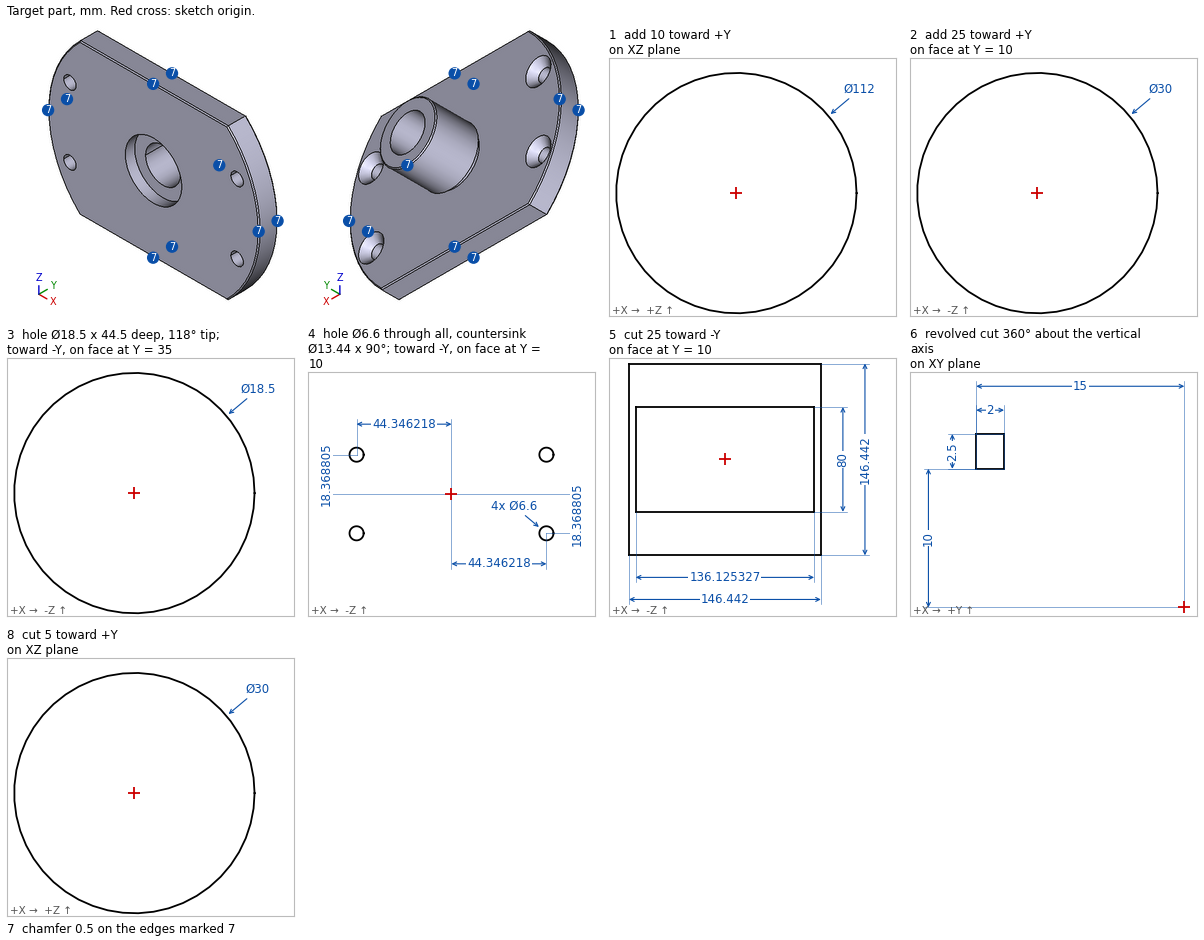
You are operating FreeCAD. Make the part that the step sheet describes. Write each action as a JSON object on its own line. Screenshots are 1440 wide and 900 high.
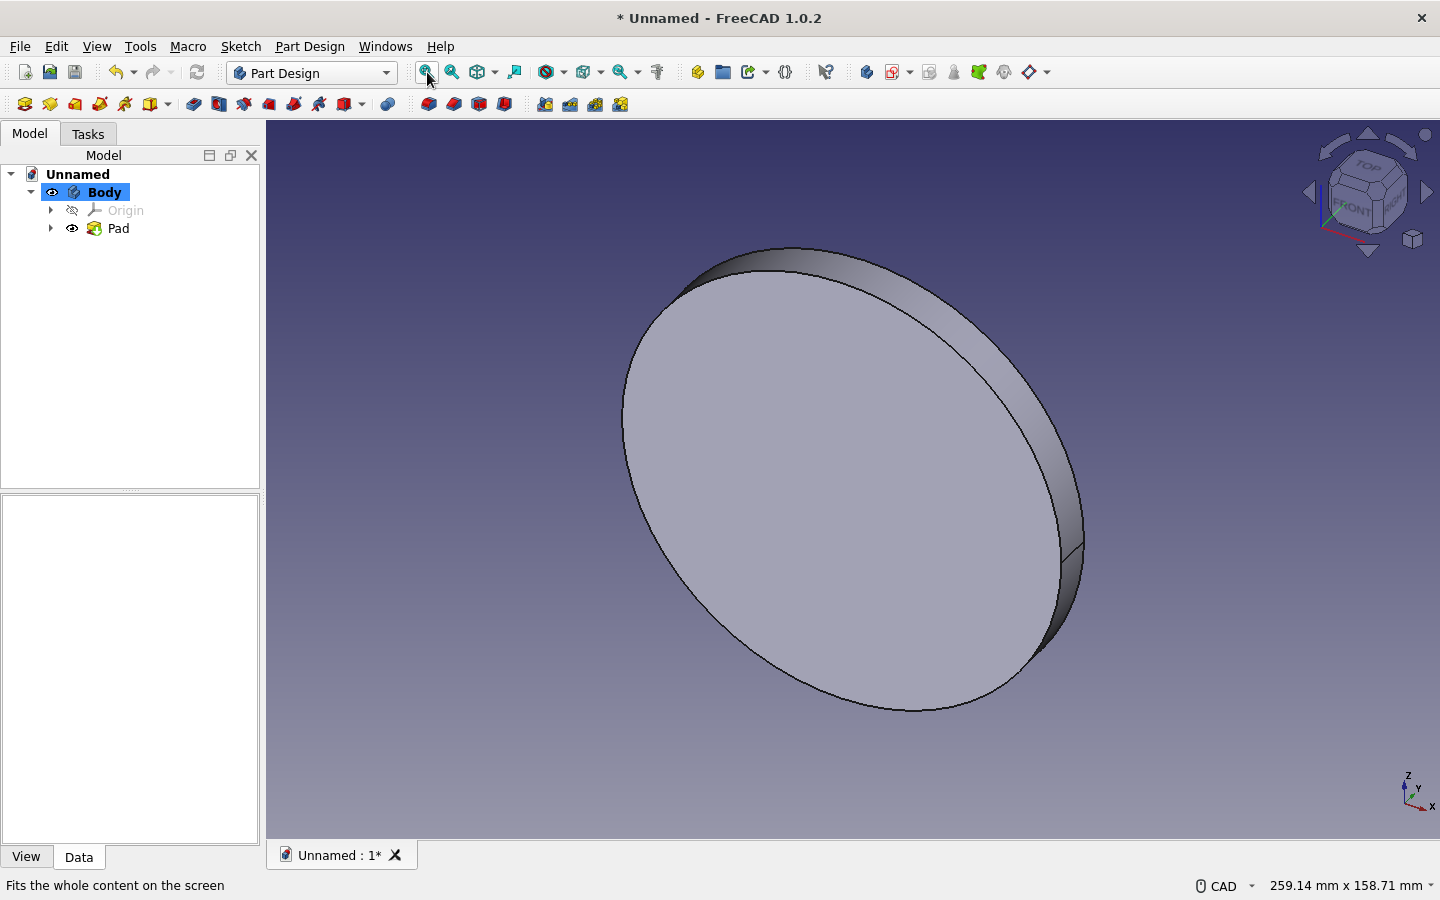
{"action": "key", "text": "4"}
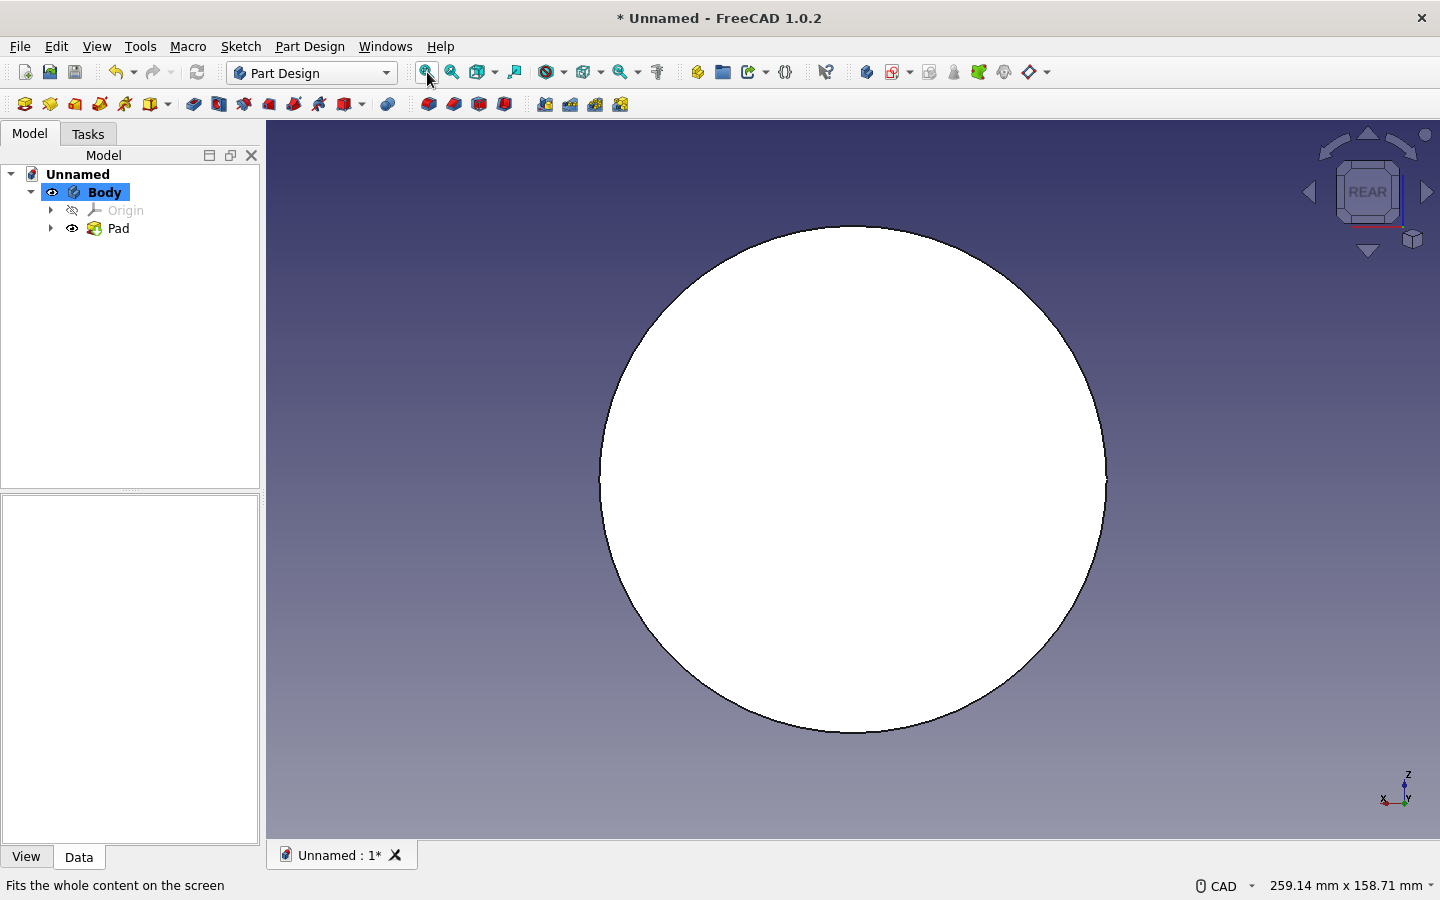
{"action": "left_click", "coordinate": [853, 478]}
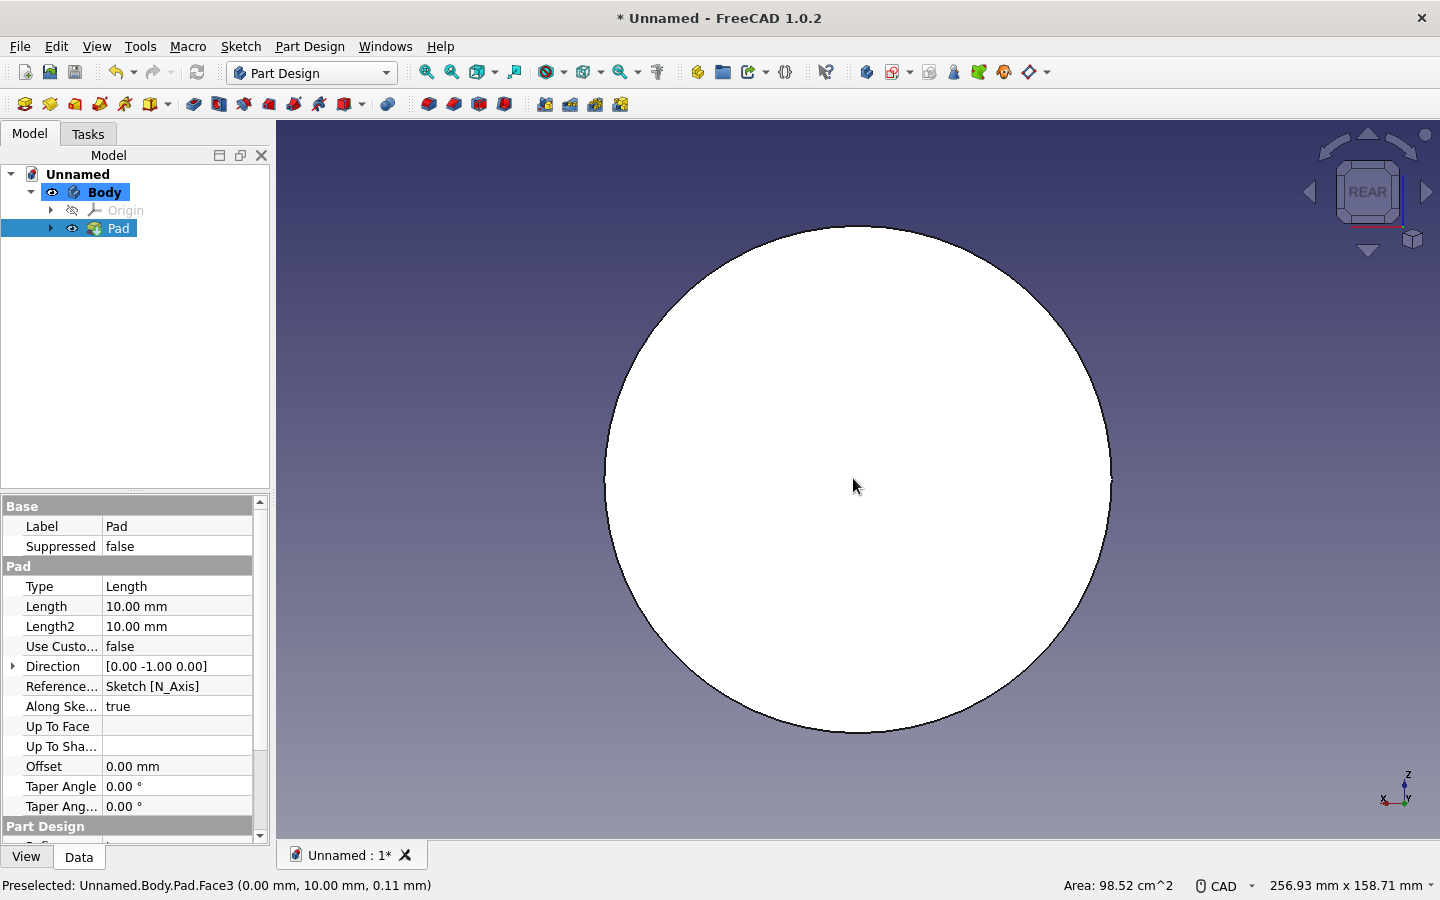
{"action": "left_click", "coordinate": [892, 72]}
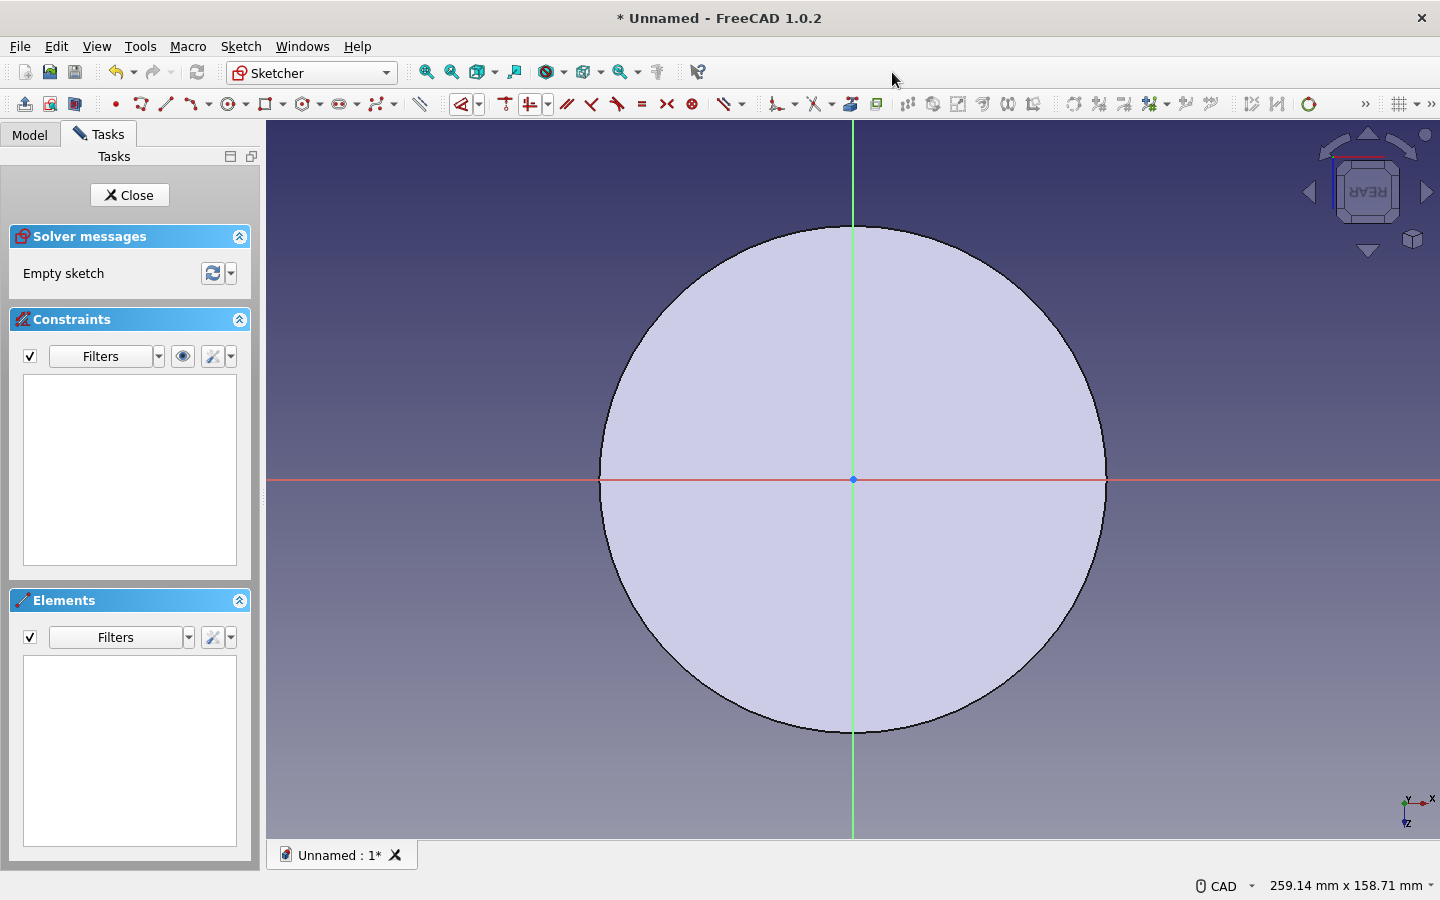
{"action": "scroll", "coordinate": [883, 480], "scroll_direction": "up", "scroll_amount": 6}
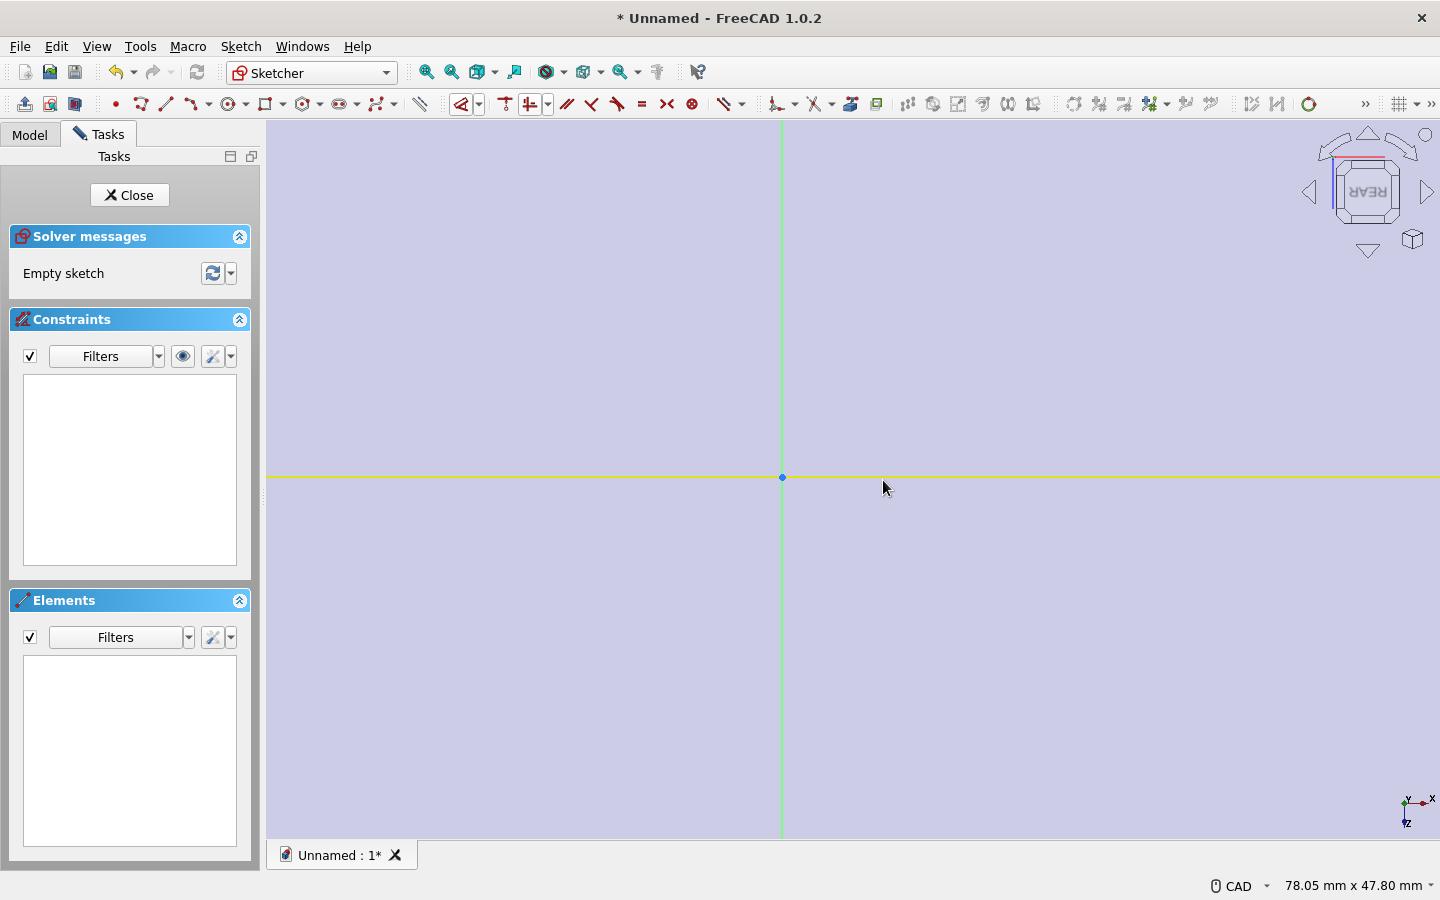
{"action": "left_click", "coordinate": [228, 104]}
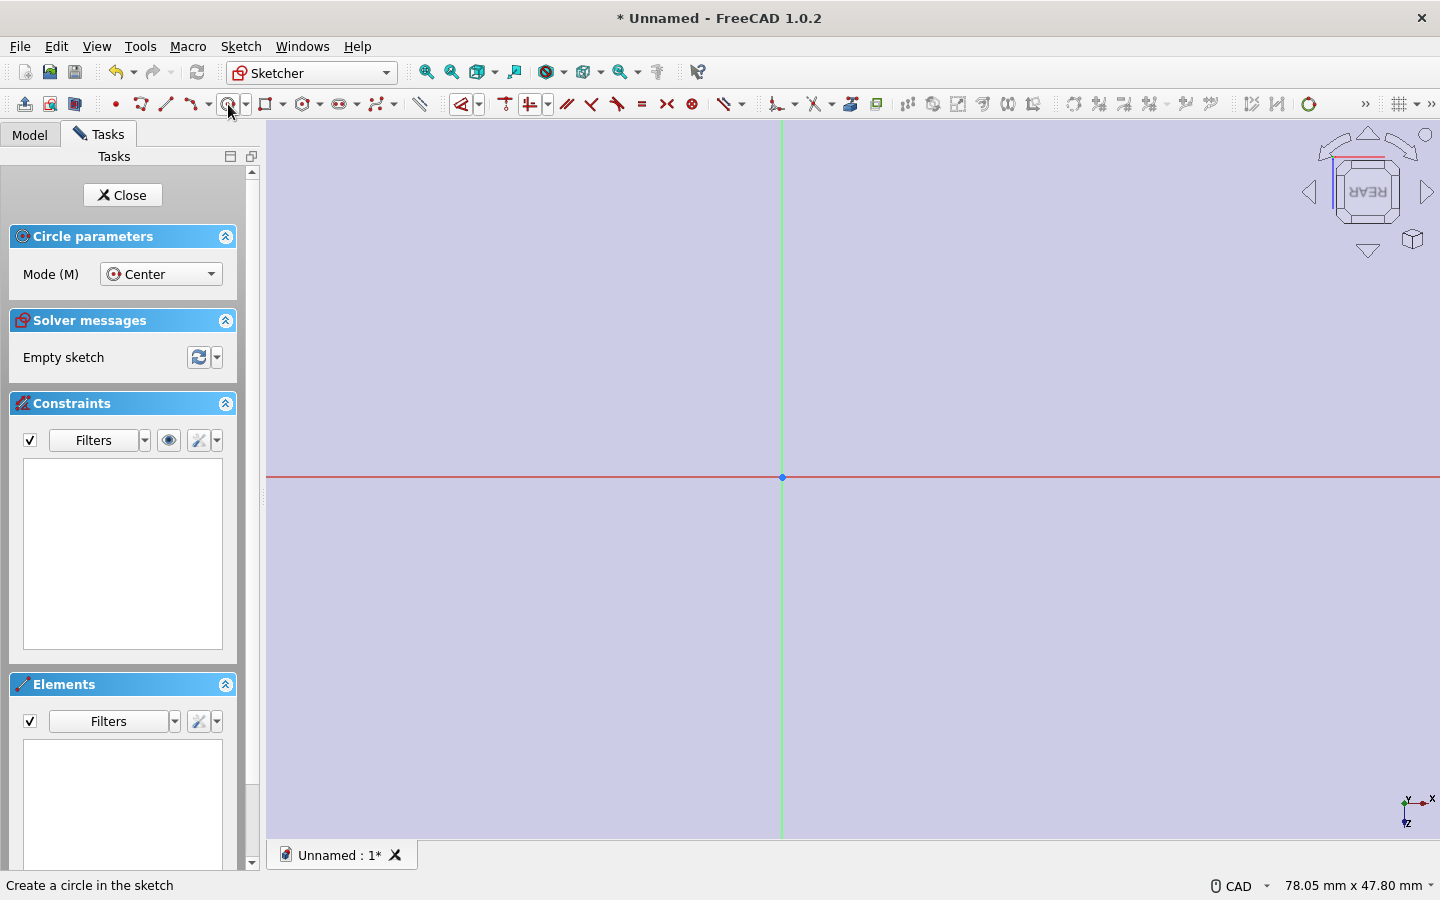
{"action": "left_click", "coordinate": [782, 477]}
{"action": "mouse_move", "coordinate": [942, 318]}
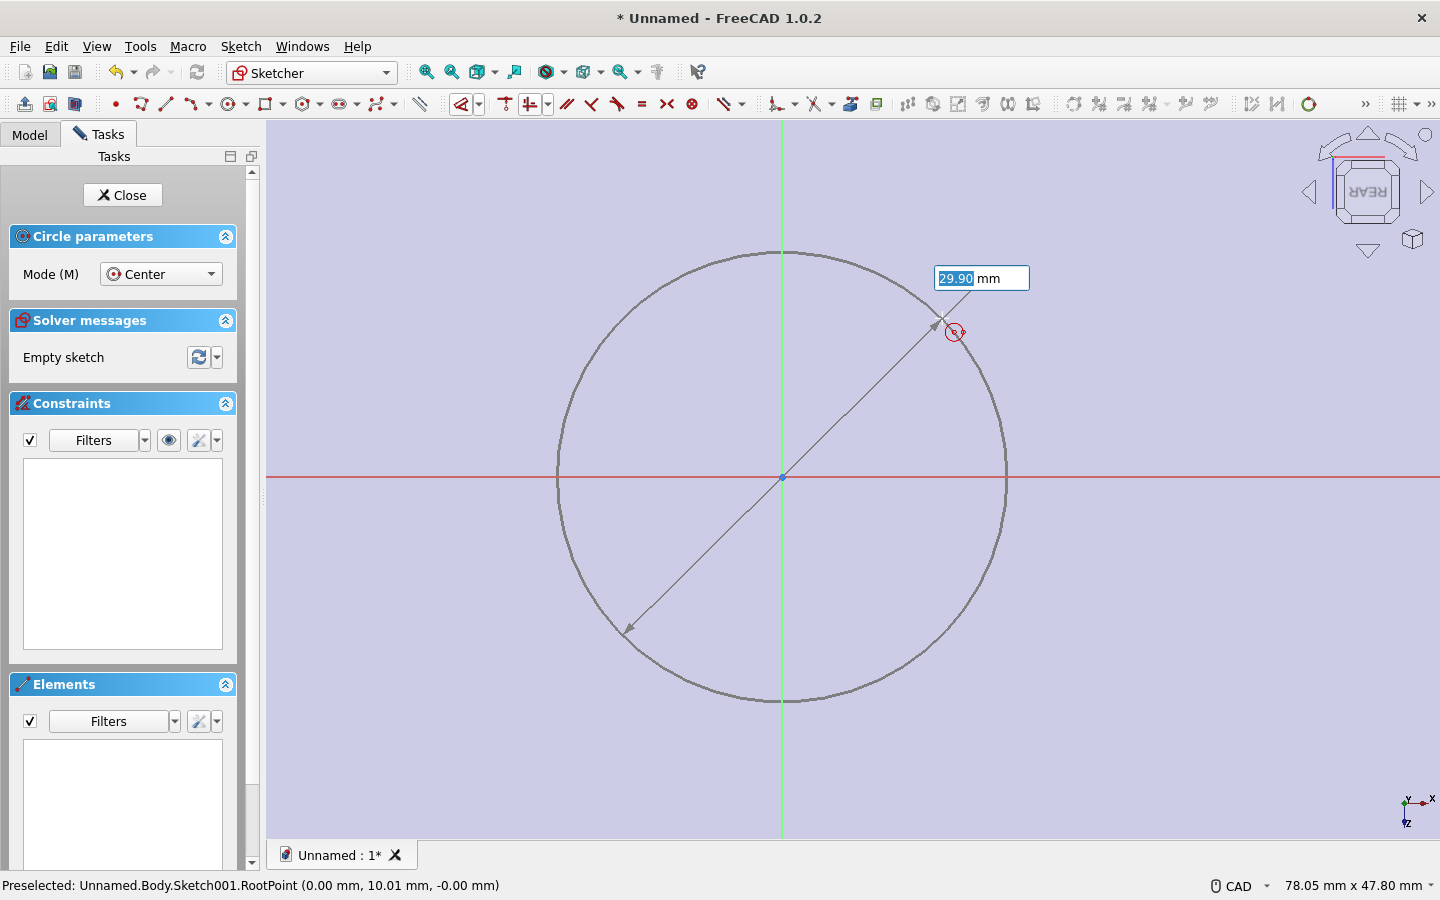
{"action": "type", "text": "30"}
{"action": "key", "text": "Return"}
{"action": "key", "text": "Escape"}